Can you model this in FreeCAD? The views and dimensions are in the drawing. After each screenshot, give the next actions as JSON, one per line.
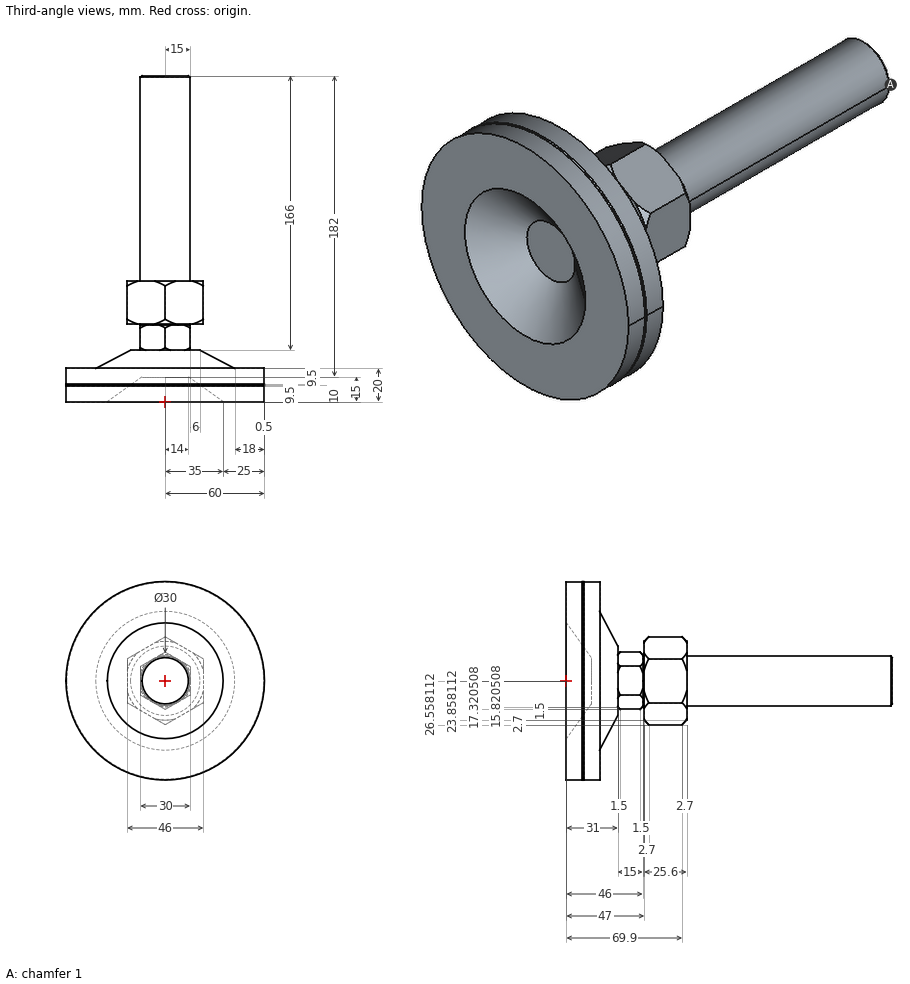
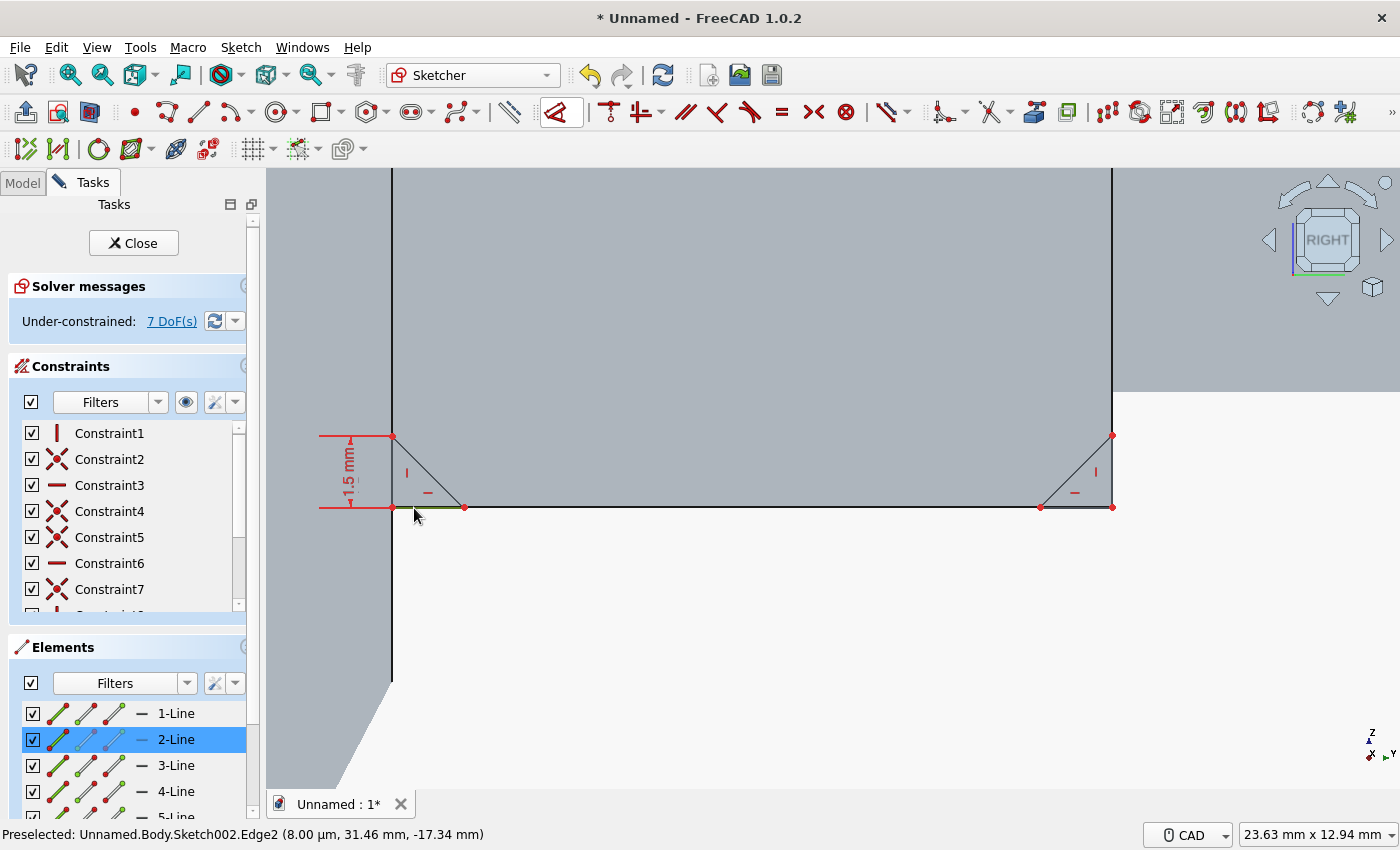
{"action": "key", "text": "l"}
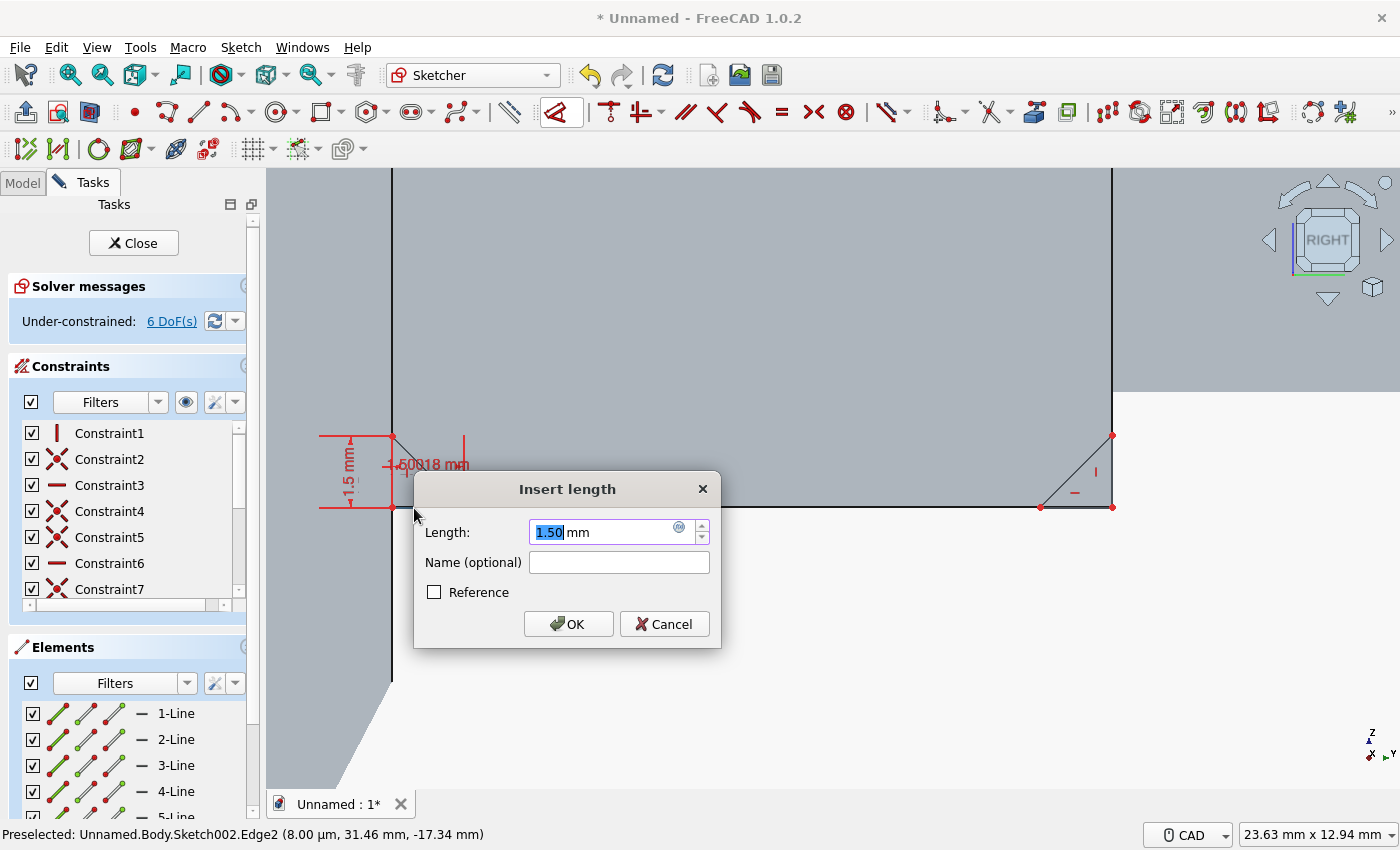
{"action": "type", "text": "1.5"}
{"action": "key", "text": "Return"}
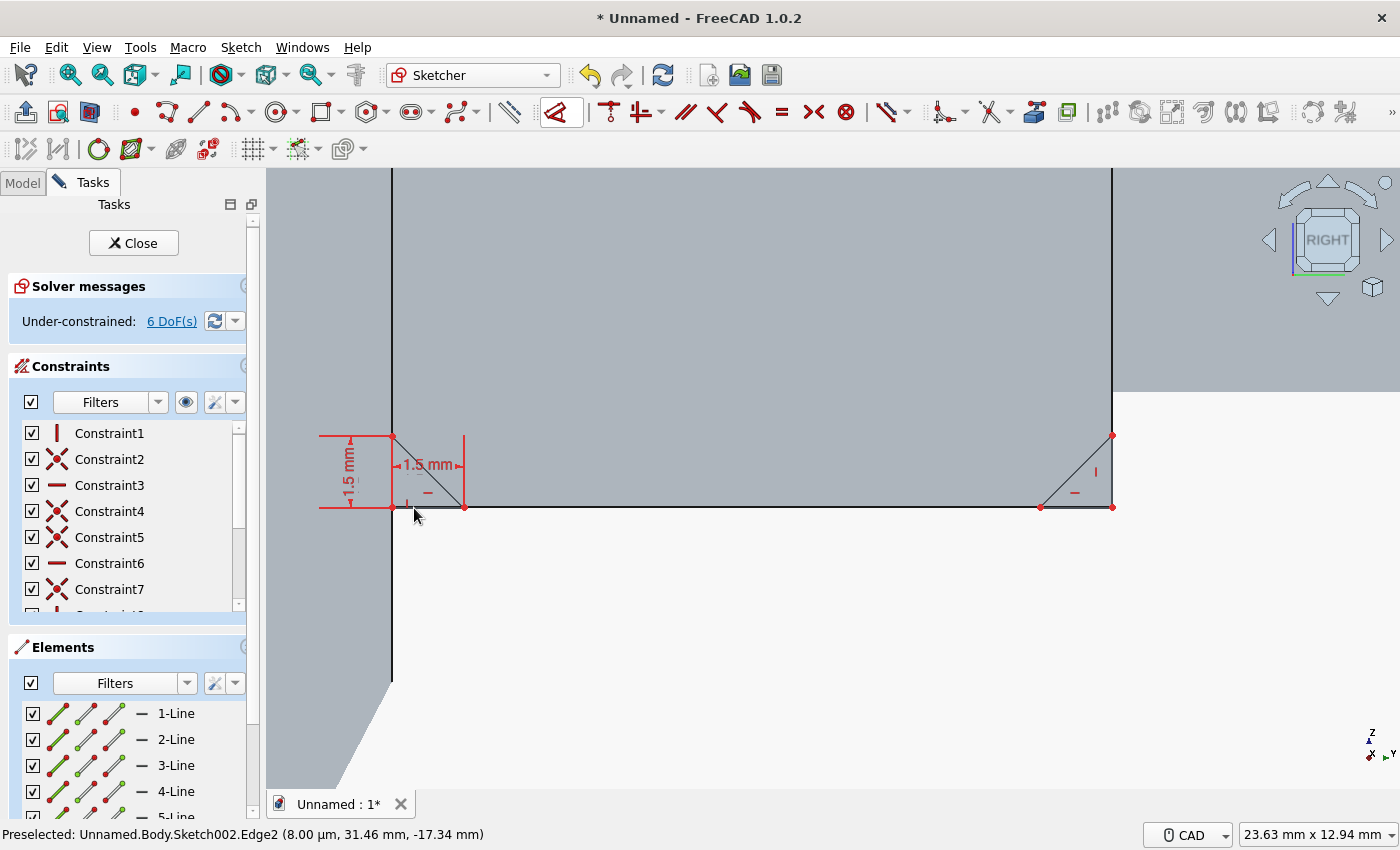
{"action": "left_click", "coordinate": [1062, 508]}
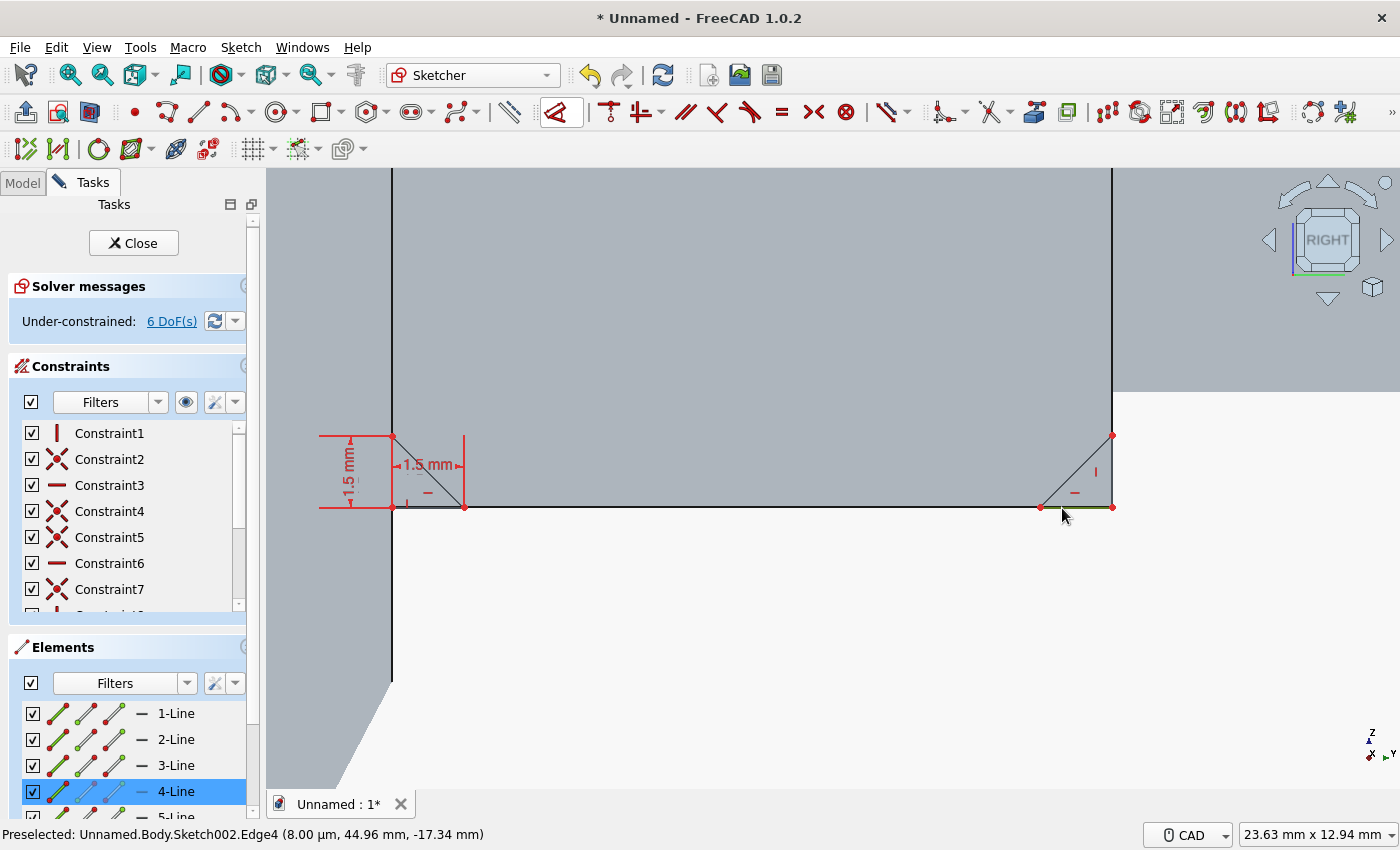
{"action": "key", "text": "l"}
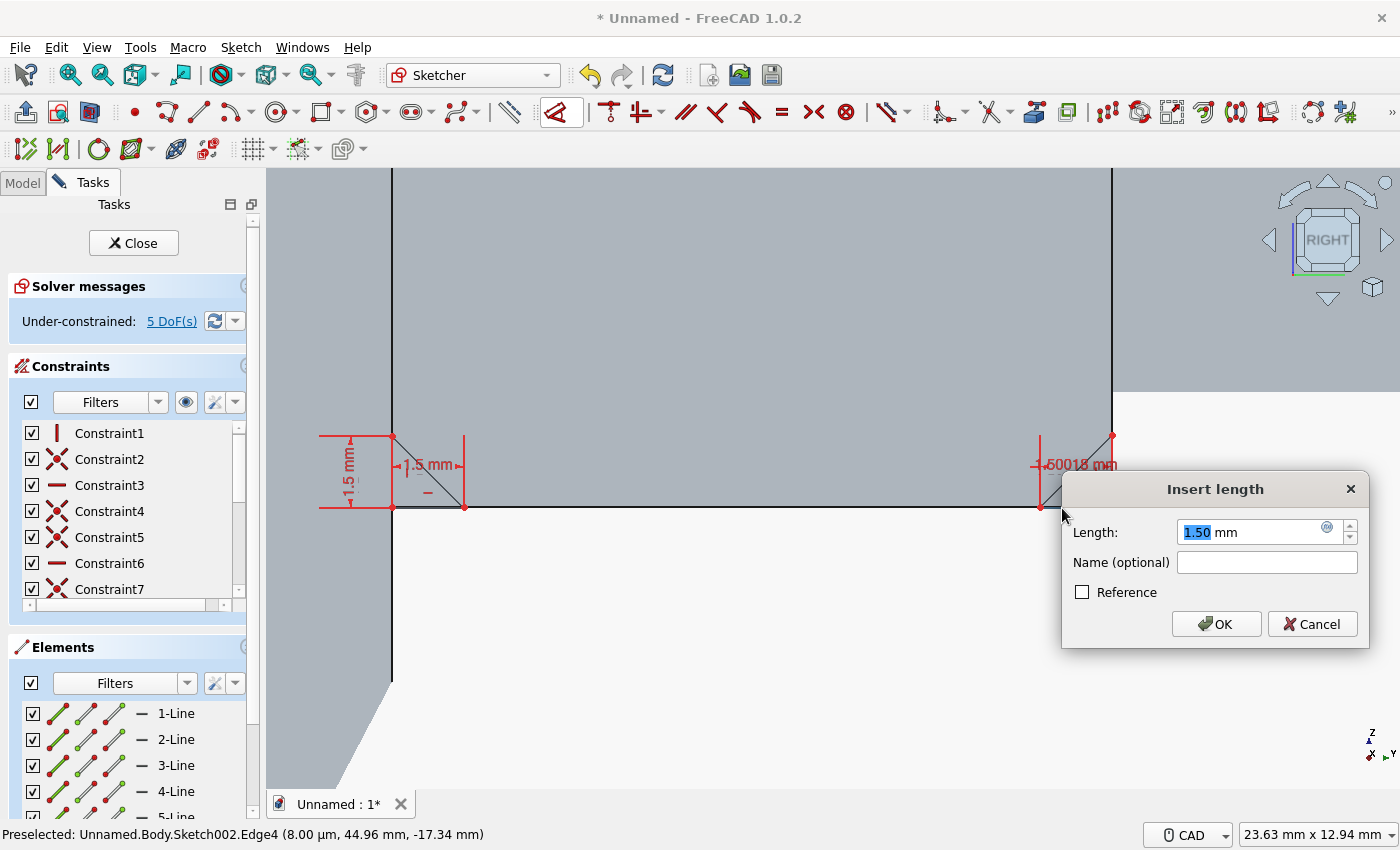
{"action": "type", "text": "1.5"}
{"action": "key", "text": "Return"}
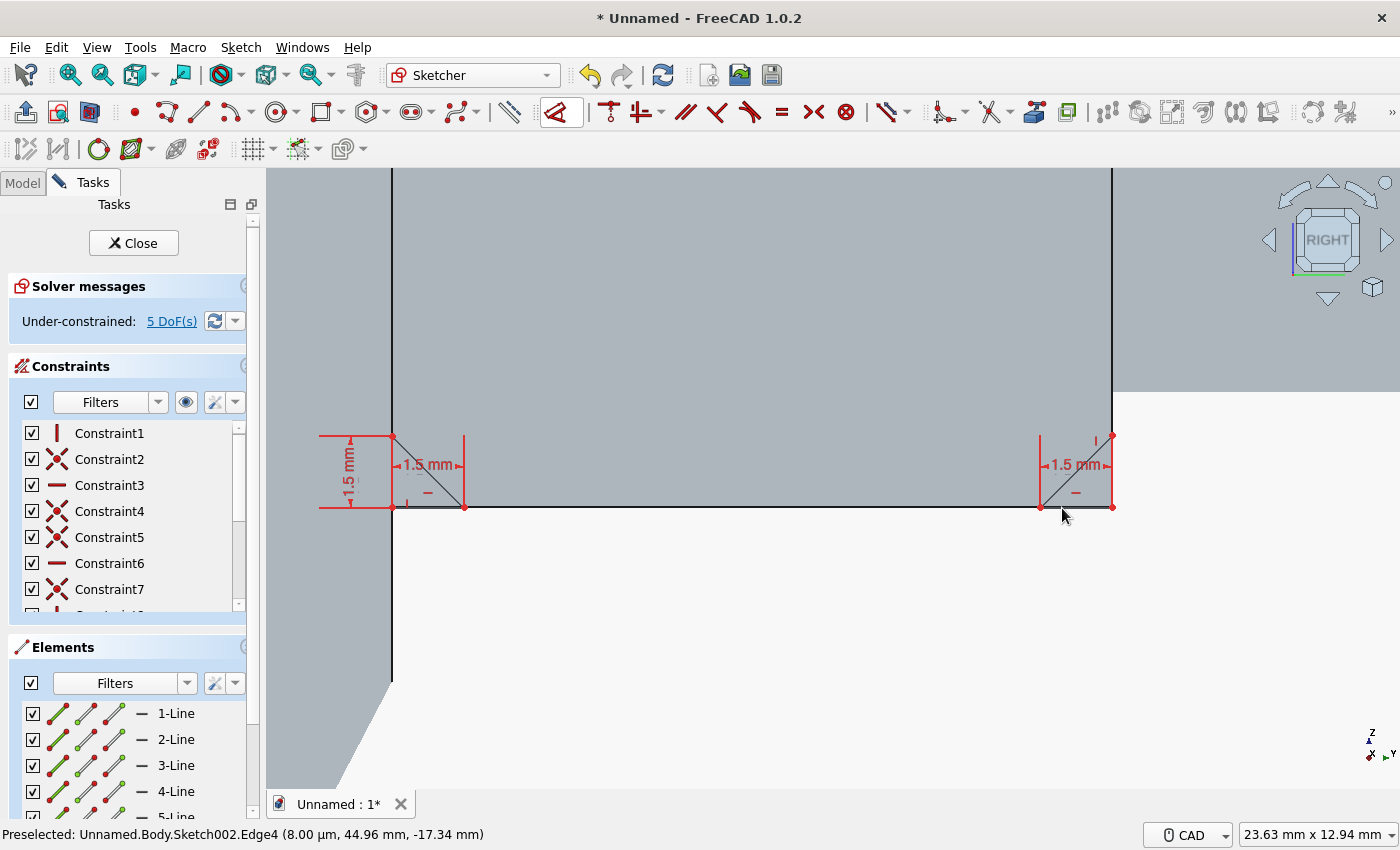
{"action": "left_click", "coordinate": [1112, 486]}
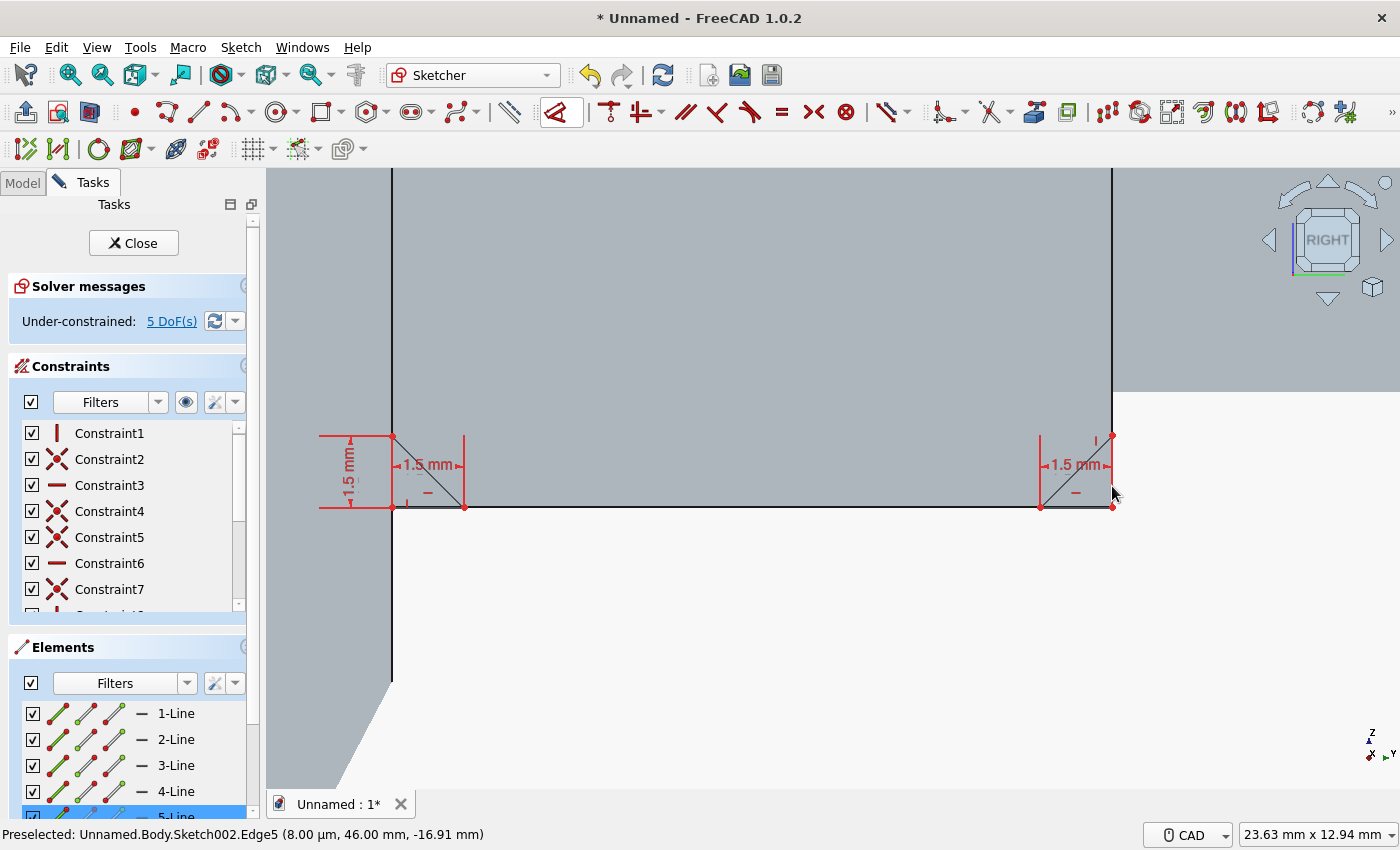
{"action": "key", "text": "i"}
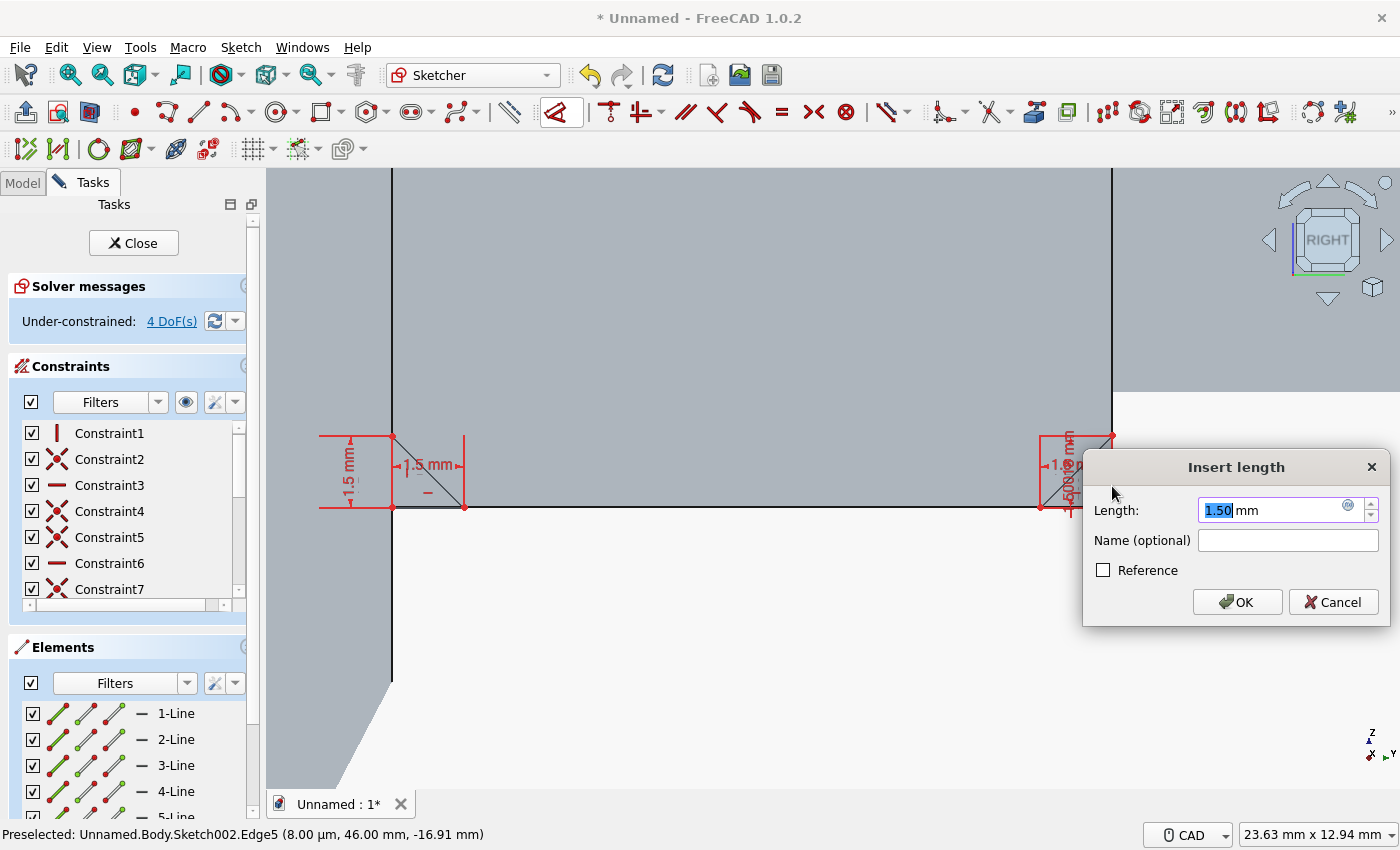
{"action": "type", "text": "1.5"}
{"action": "key", "text": "Return"}